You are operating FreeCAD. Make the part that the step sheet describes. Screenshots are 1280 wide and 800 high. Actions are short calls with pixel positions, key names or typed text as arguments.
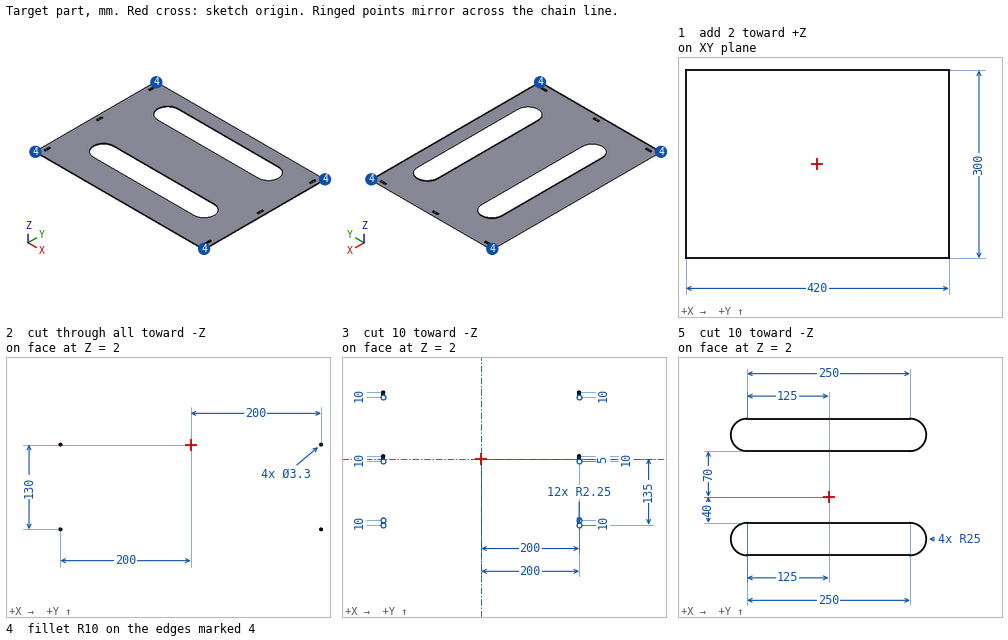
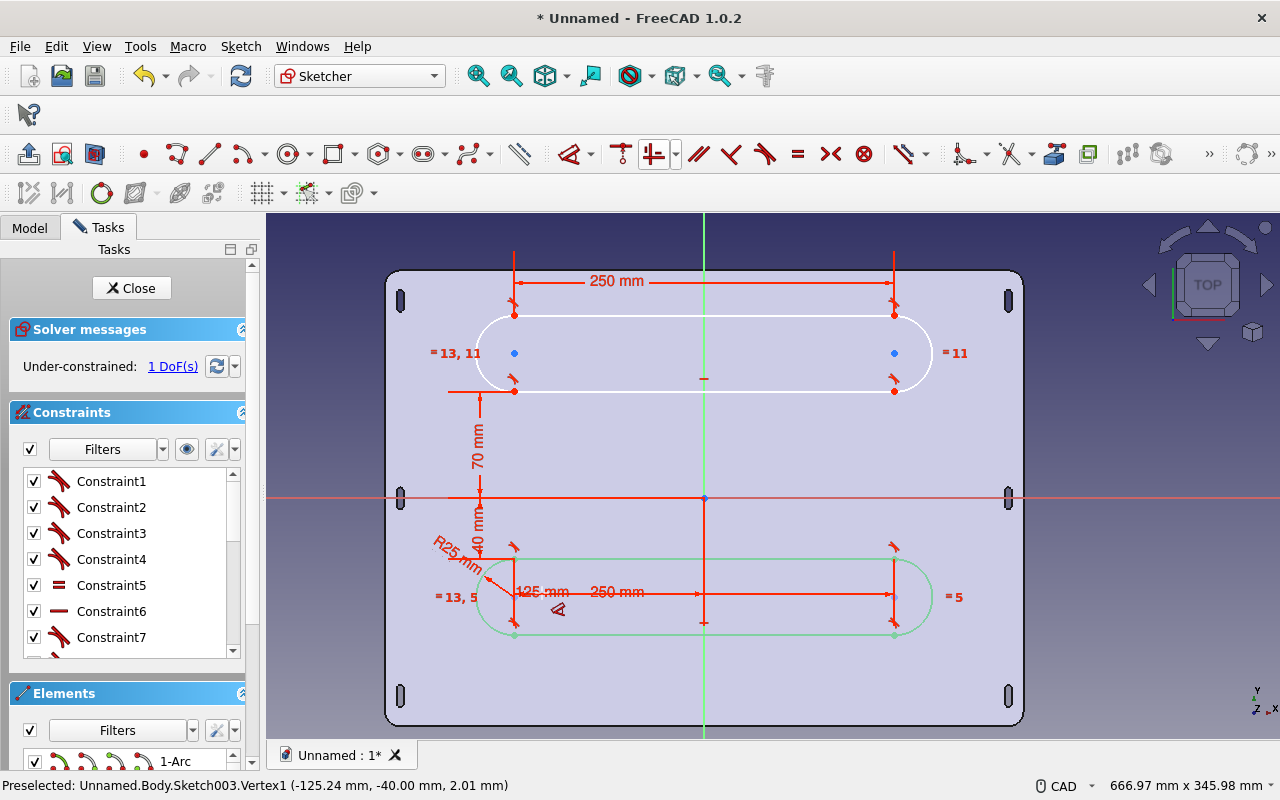
click(514, 316)
click(543, 282)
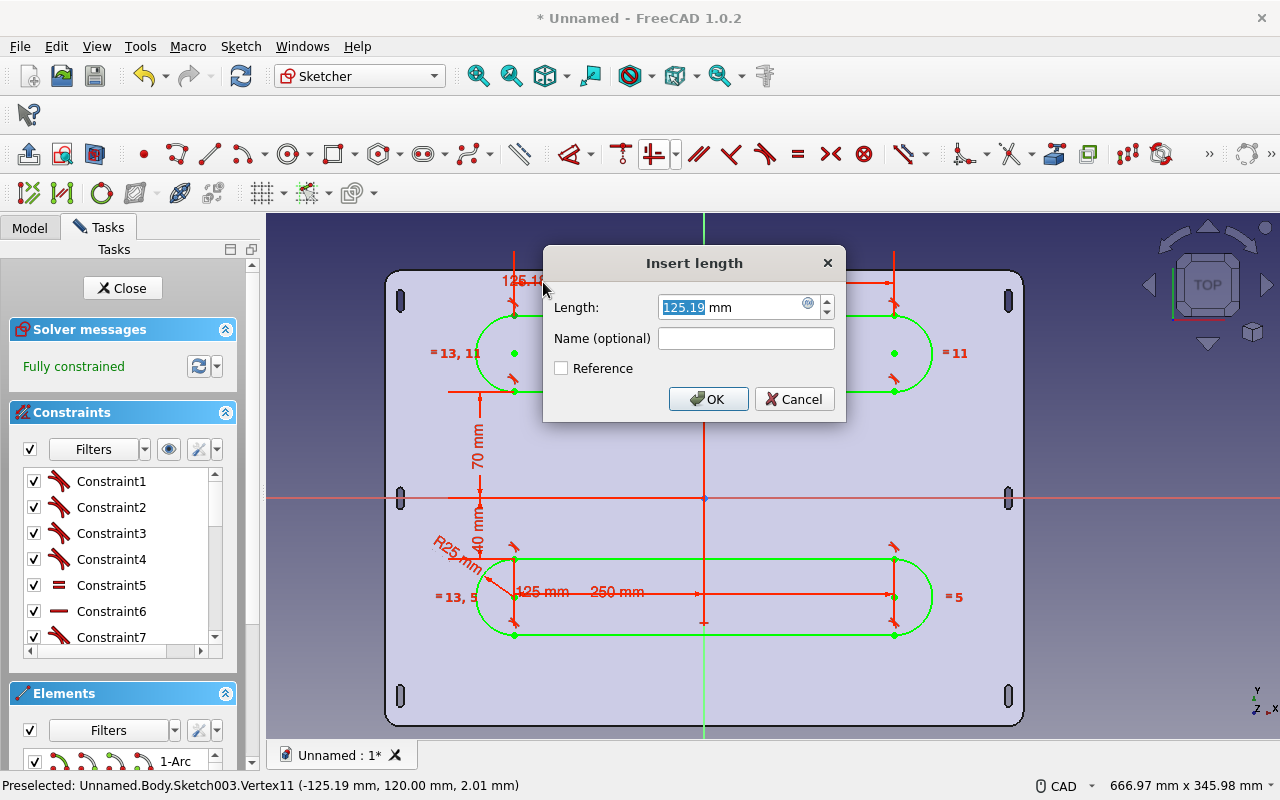
text(125)
key(Return)
key(Escape)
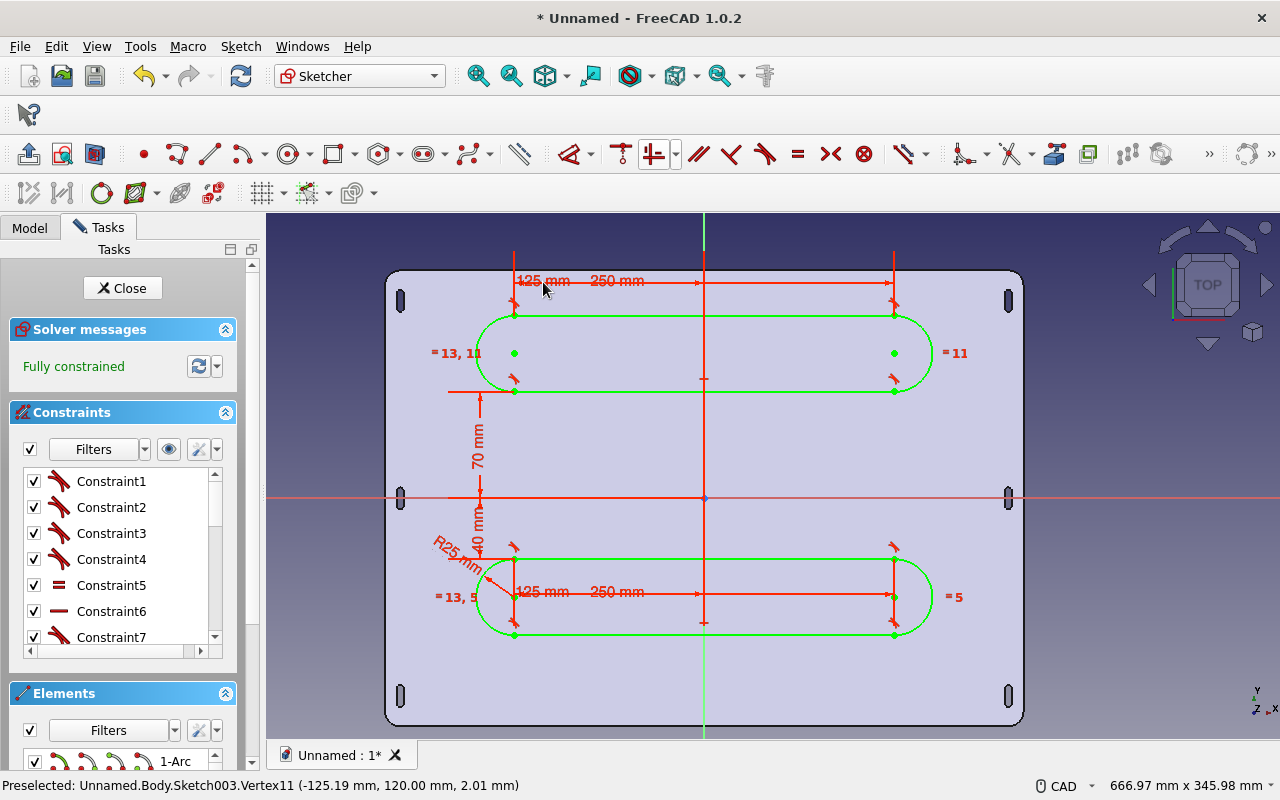
click(123, 288)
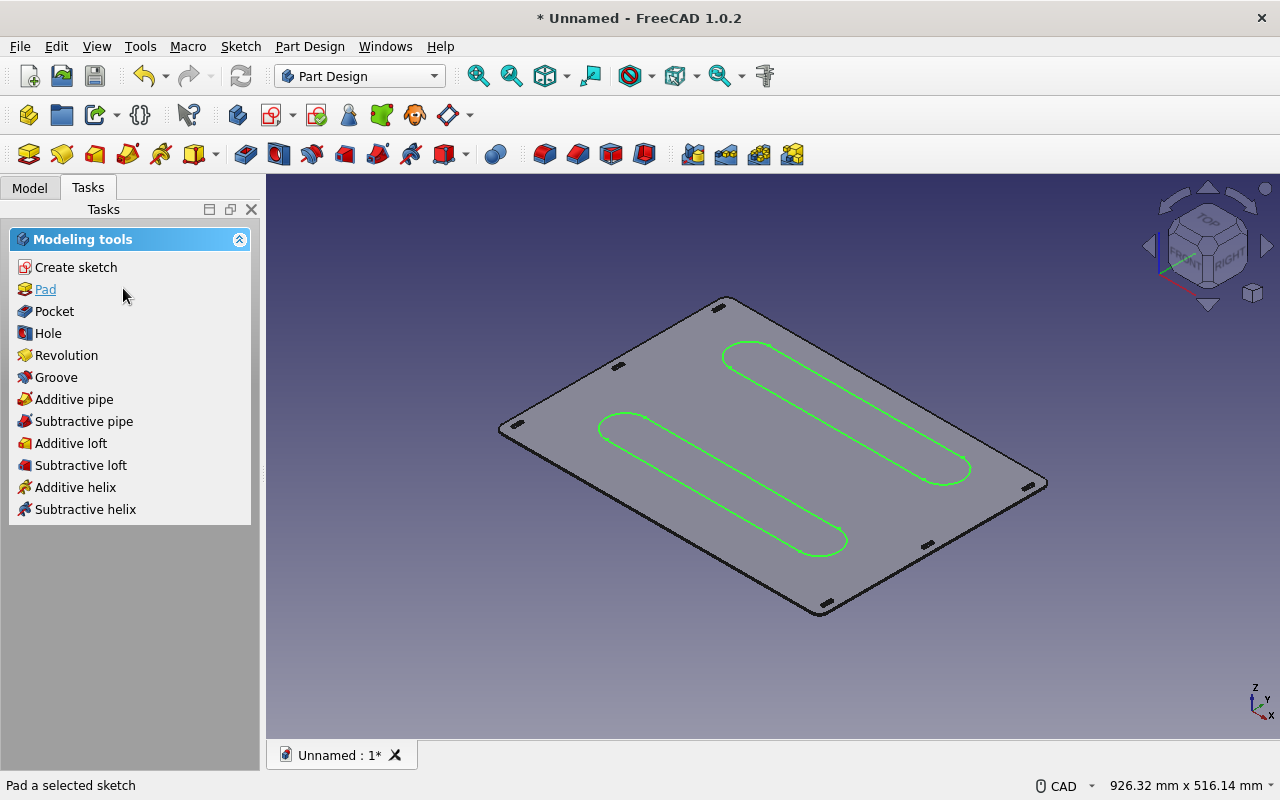
click(246, 154)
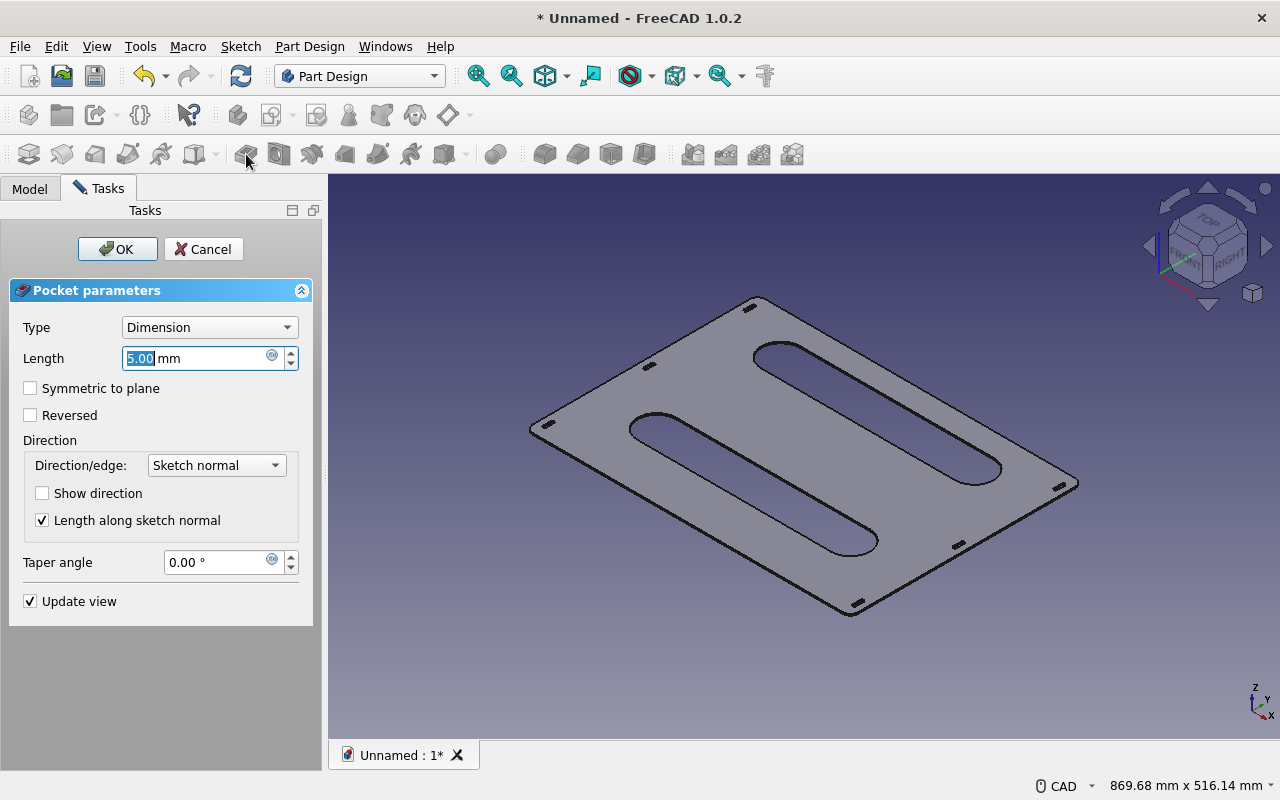
text(10)
key(Tab)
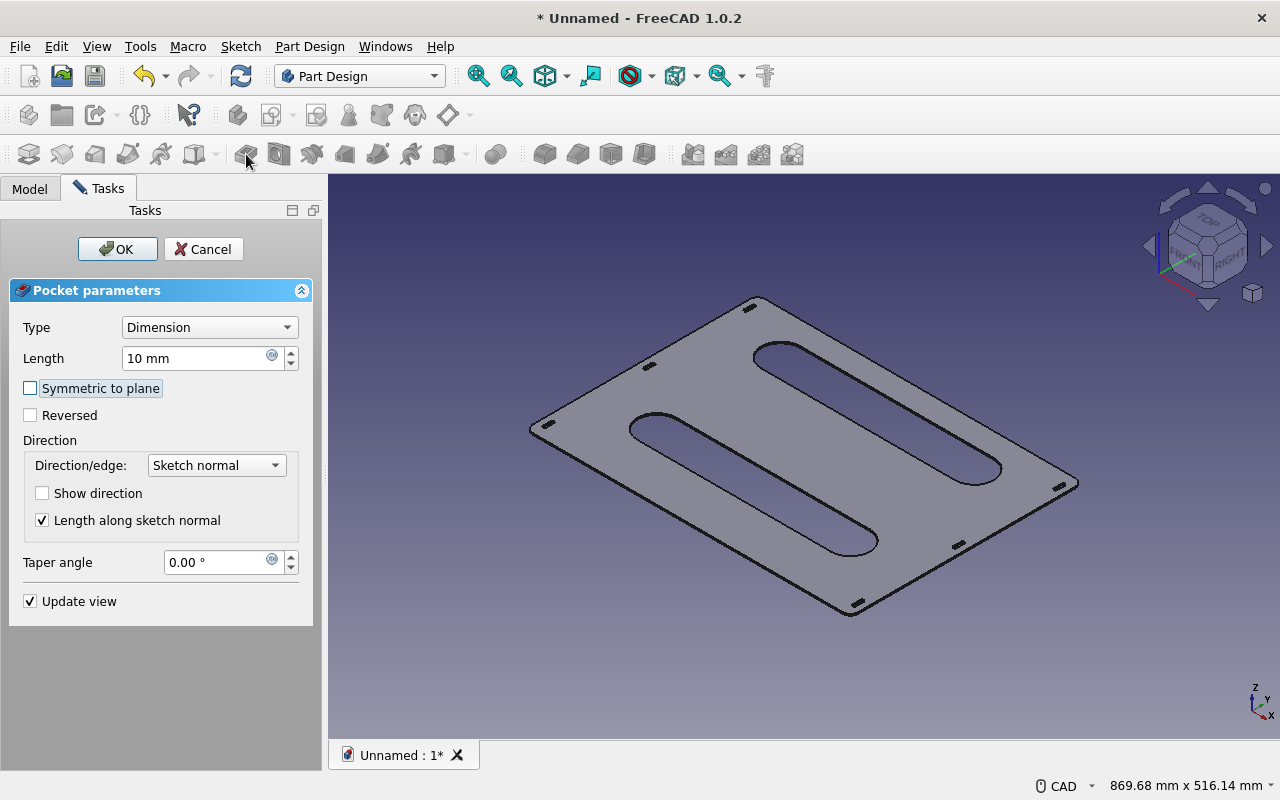
click(118, 249)